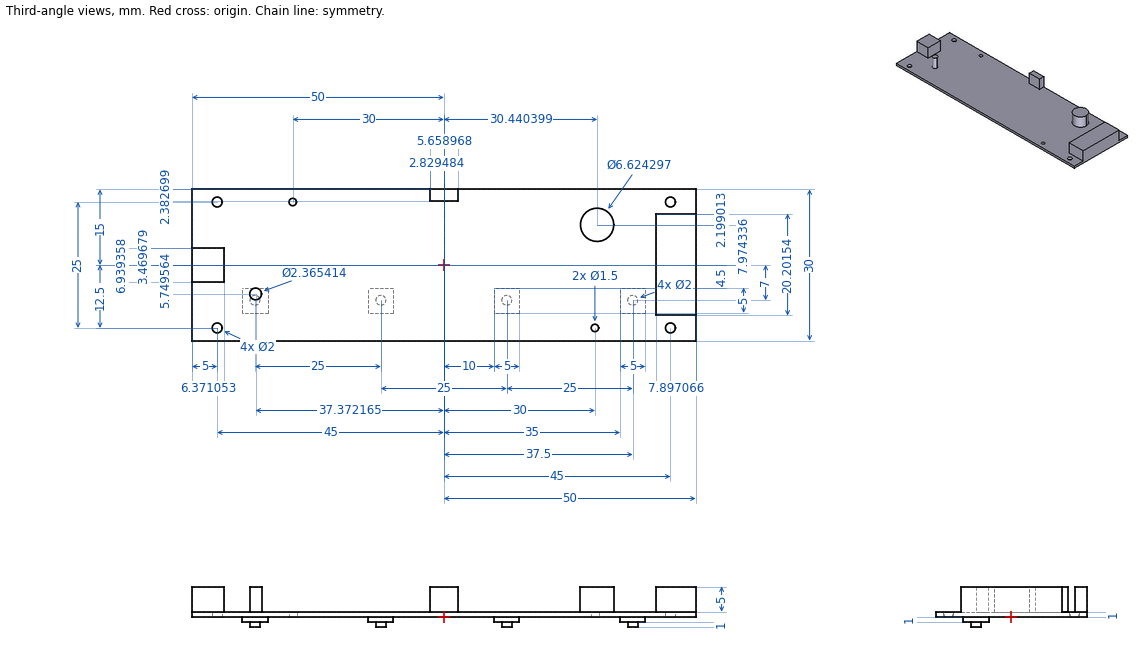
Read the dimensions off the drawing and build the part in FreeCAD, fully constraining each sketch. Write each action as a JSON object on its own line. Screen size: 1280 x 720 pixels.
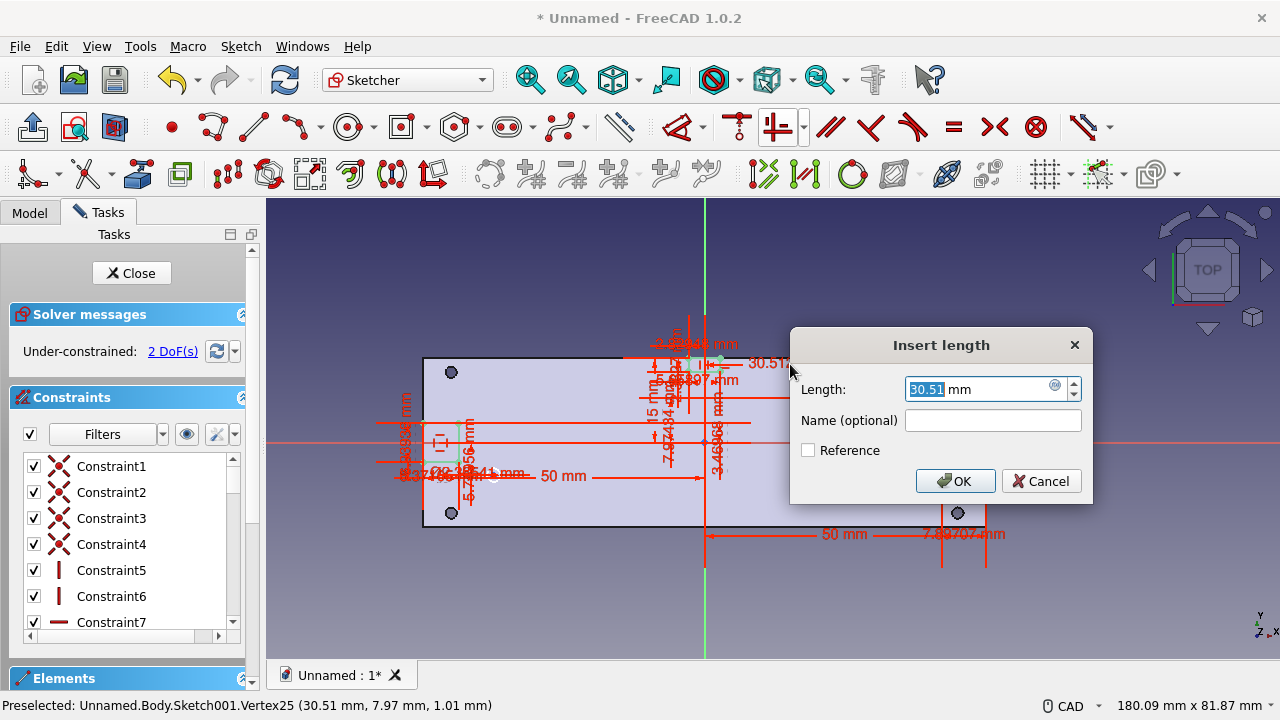
{"action": "type", "text": "30.440399"}
{"action": "key", "text": "Return"}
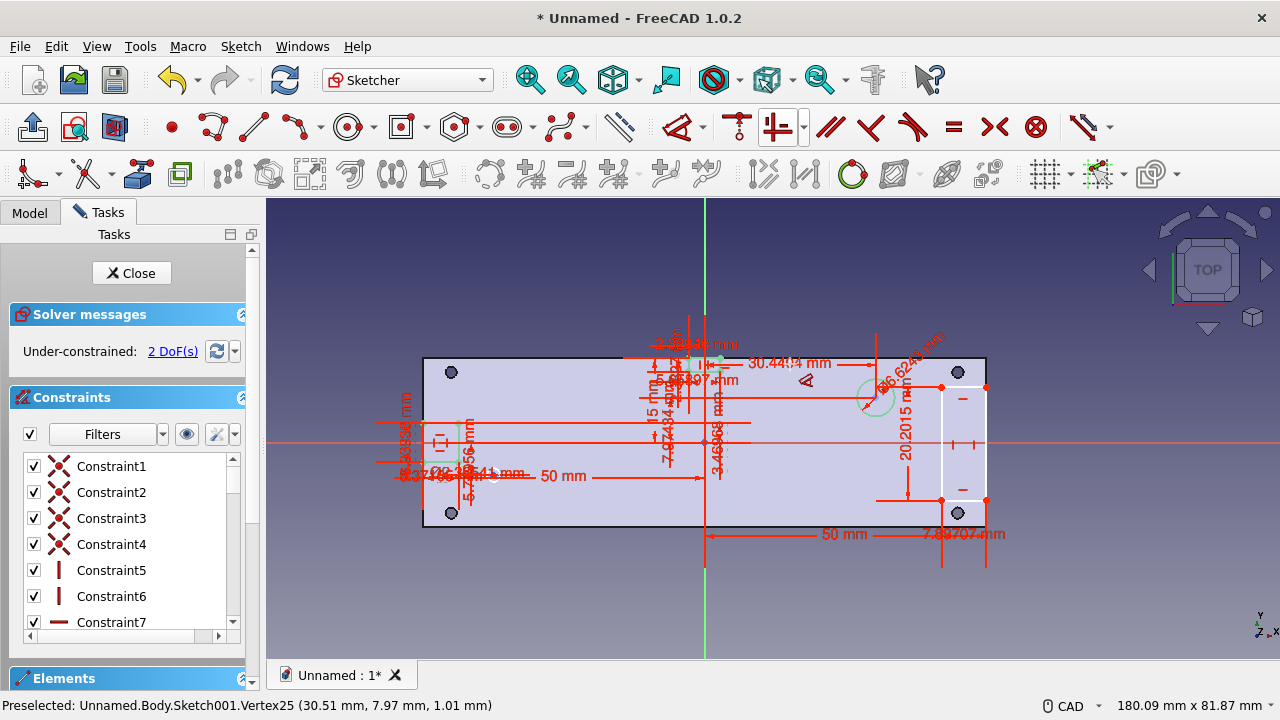
{"action": "left_click", "coordinate": [494, 475]}
{"action": "left_click", "coordinate": [599, 509]}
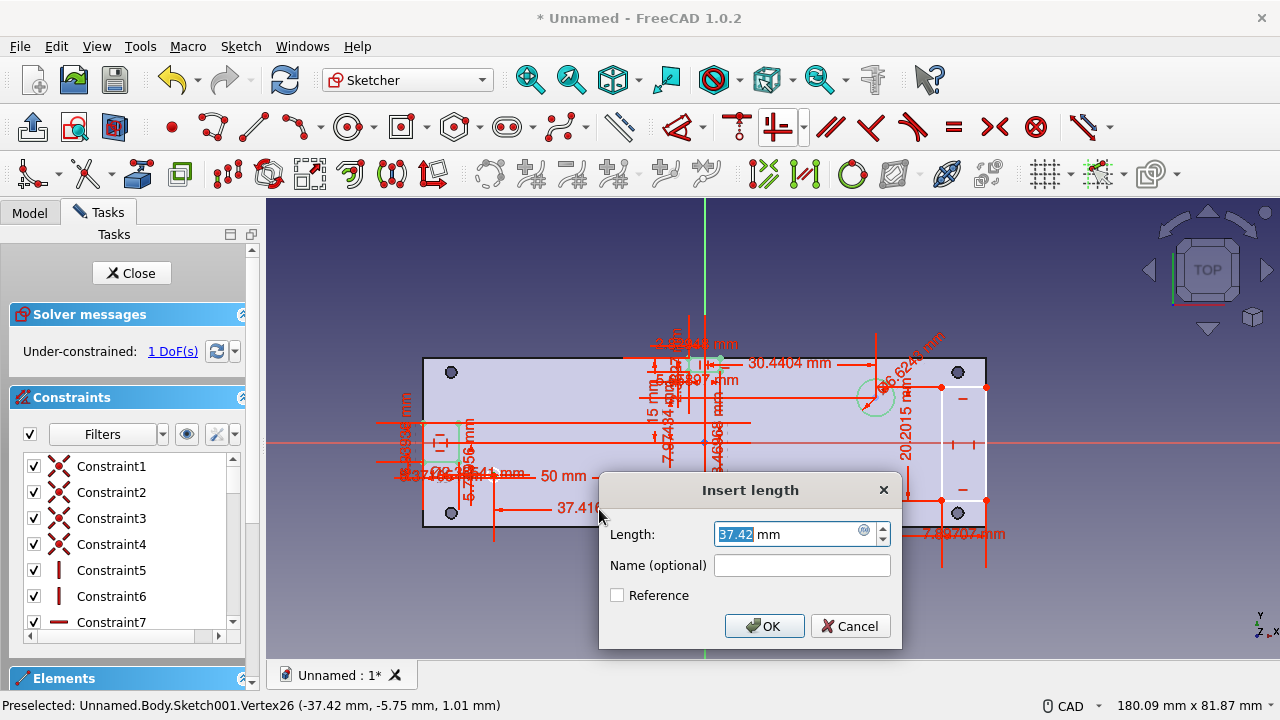
{"action": "type", "text": "37.372165"}
{"action": "key", "text": "Return"}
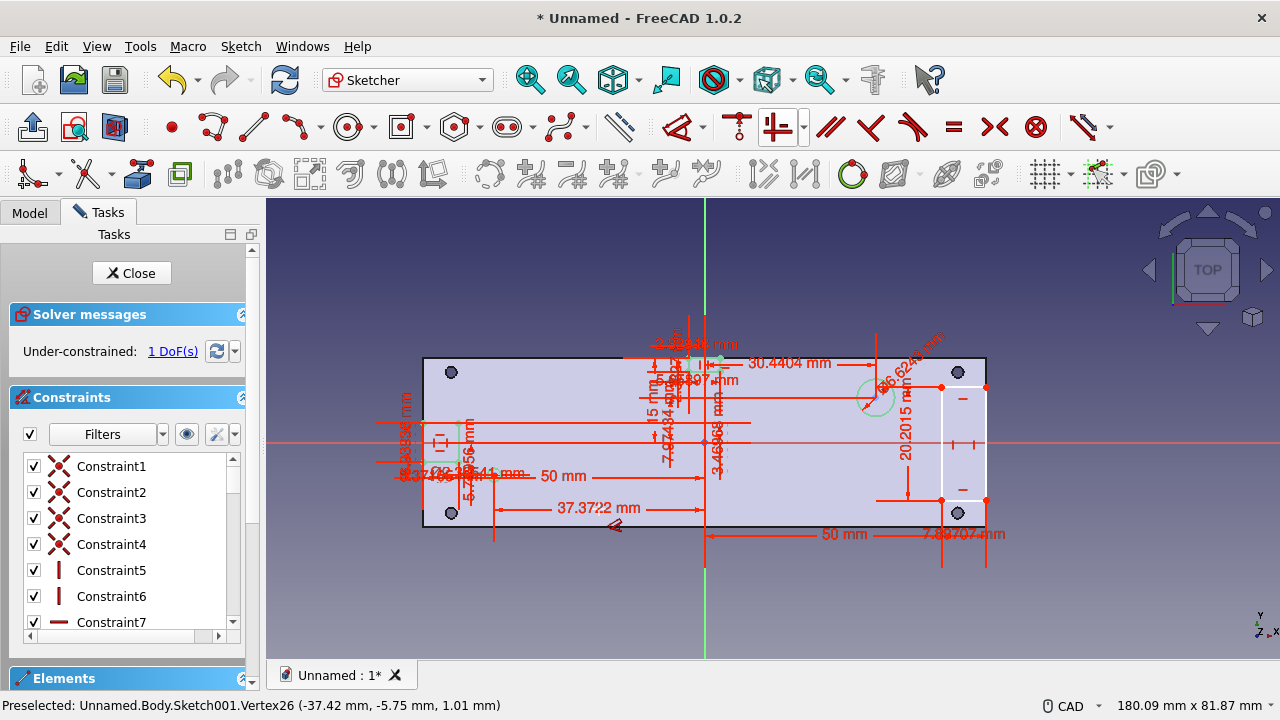
{"action": "scroll", "coordinate": [942, 387], "scroll_direction": "up", "scroll_amount": 6}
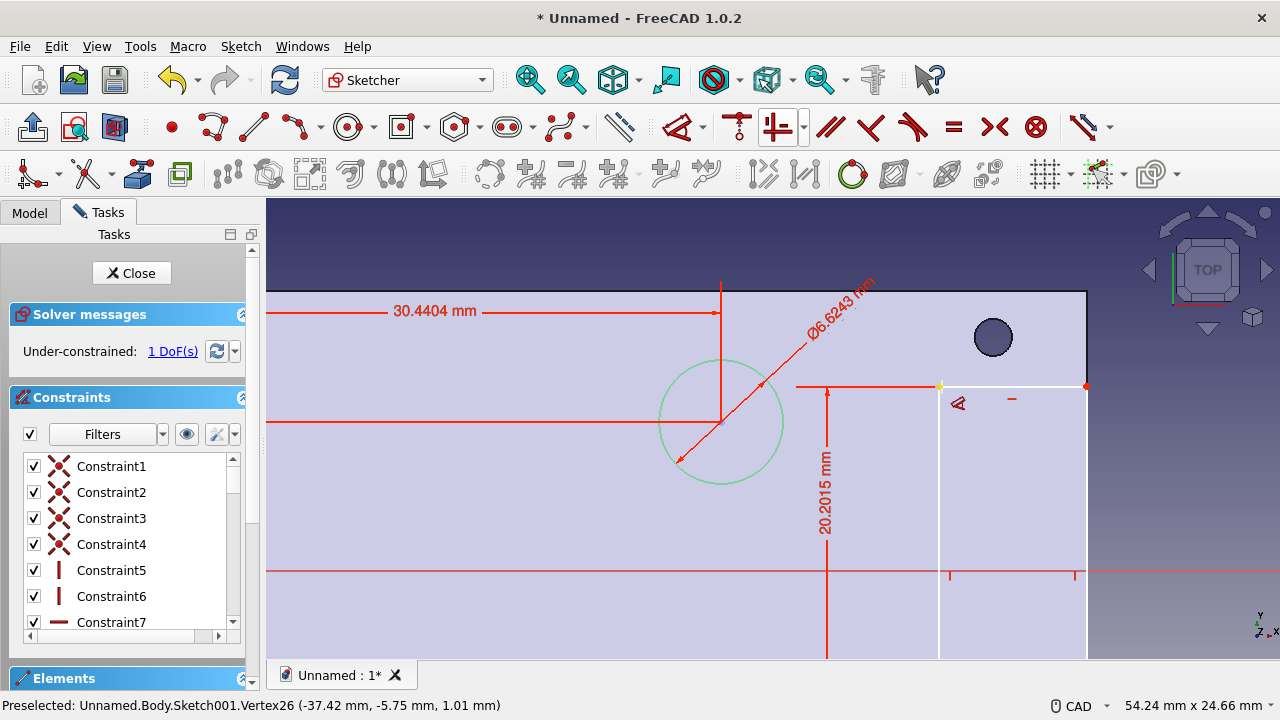
{"action": "left_click", "coordinate": [939, 387]}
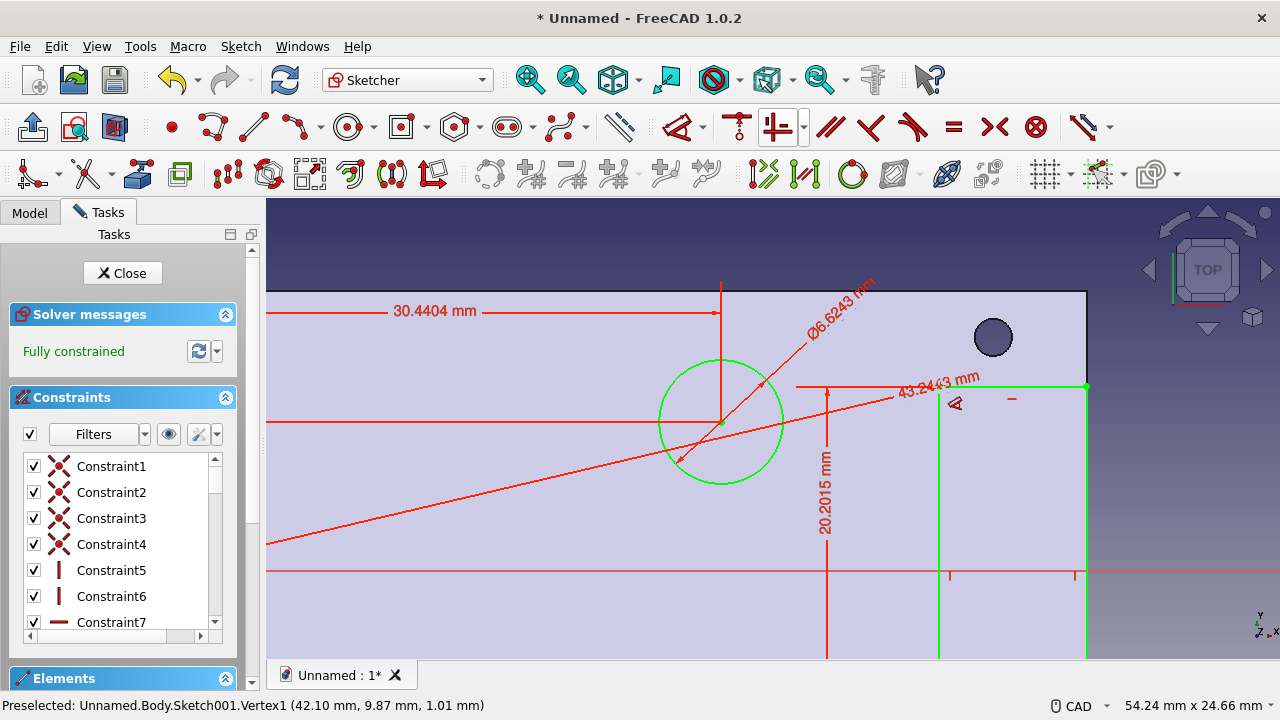
{"action": "left_click", "coordinate": [721, 422]}
{"action": "left_click", "coordinate": [973, 404]}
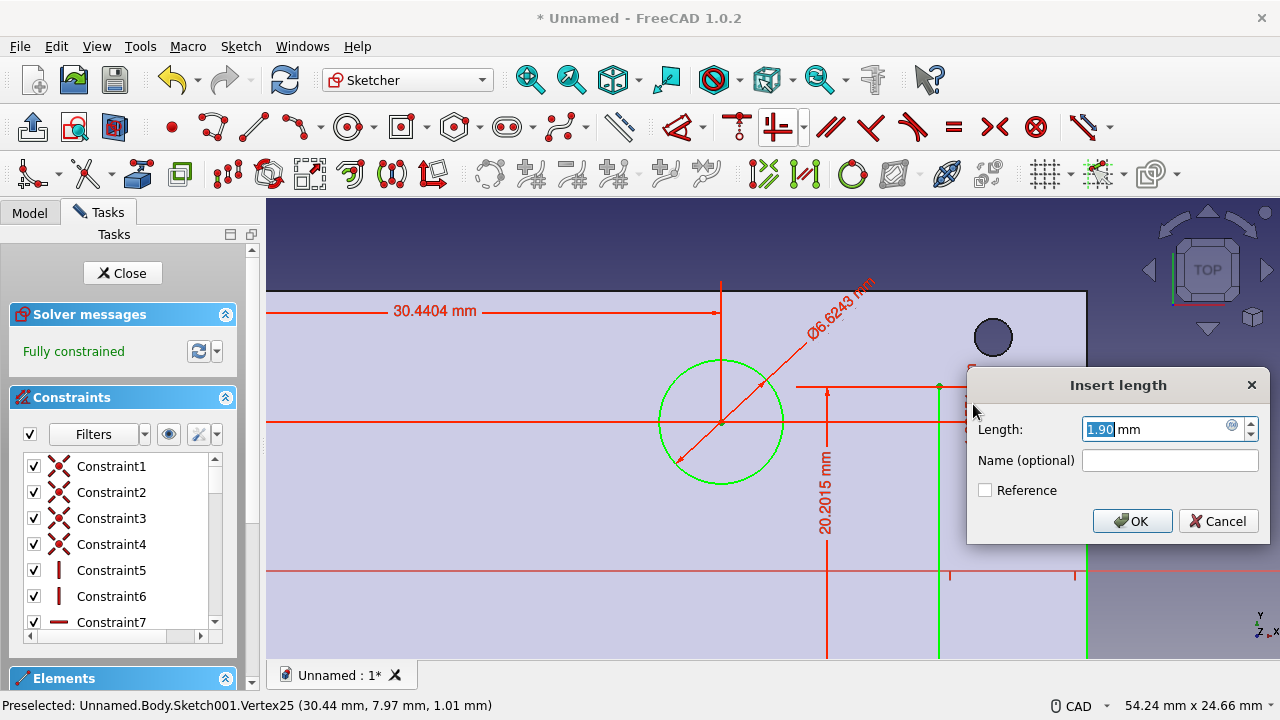
{"action": "type", "text": "2.199013"}
{"action": "key", "text": "Return"}
{"action": "key", "text": "Escape"}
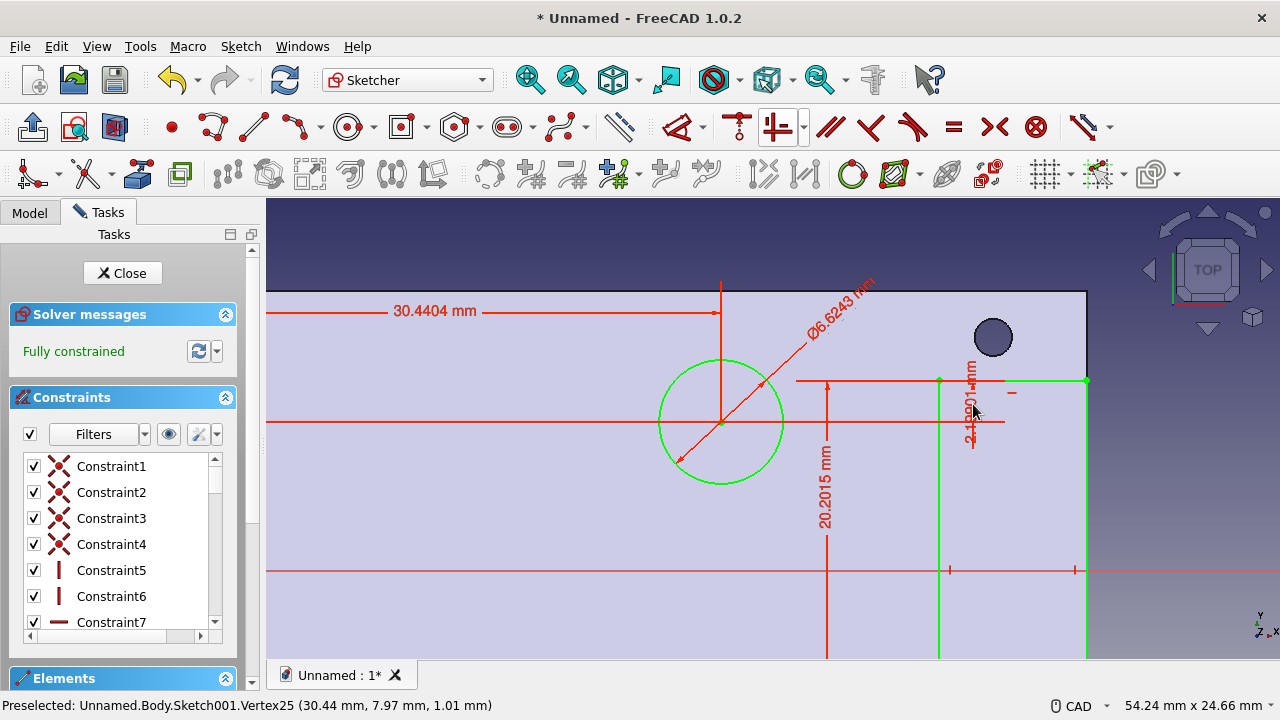
{"action": "left_click", "coordinate": [123, 273]}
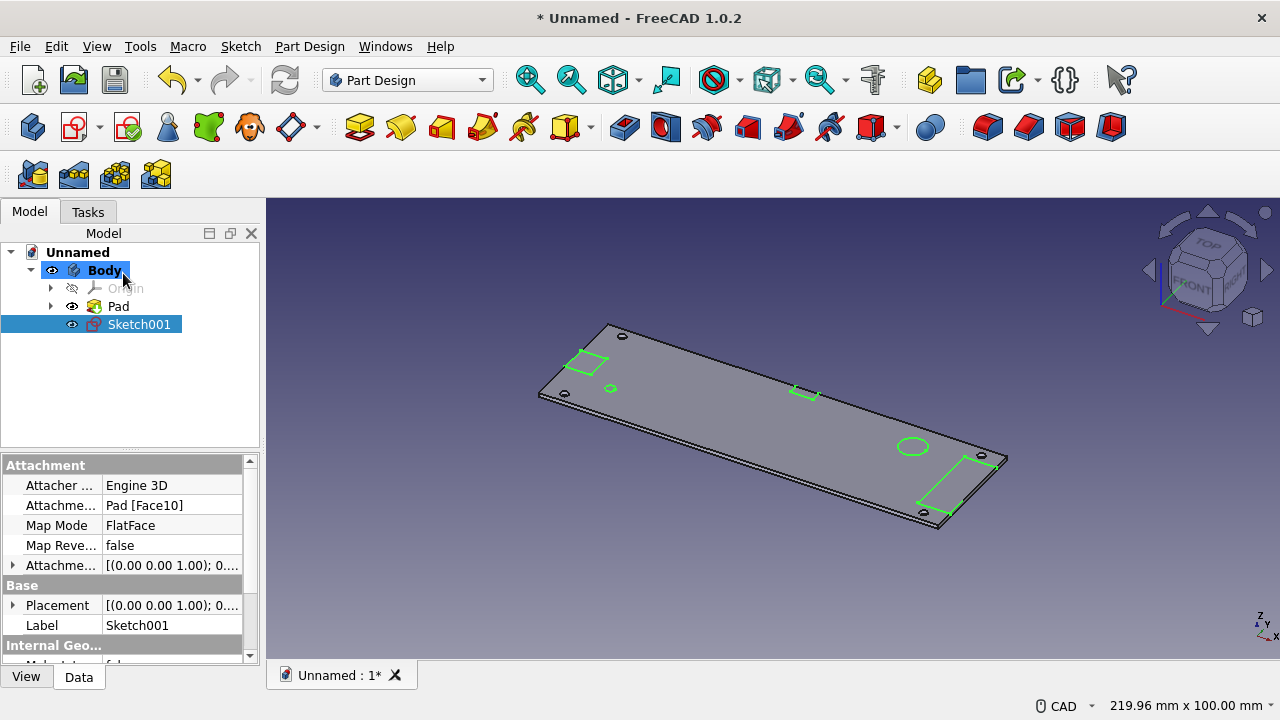
{"action": "left_click", "coordinate": [360, 128]}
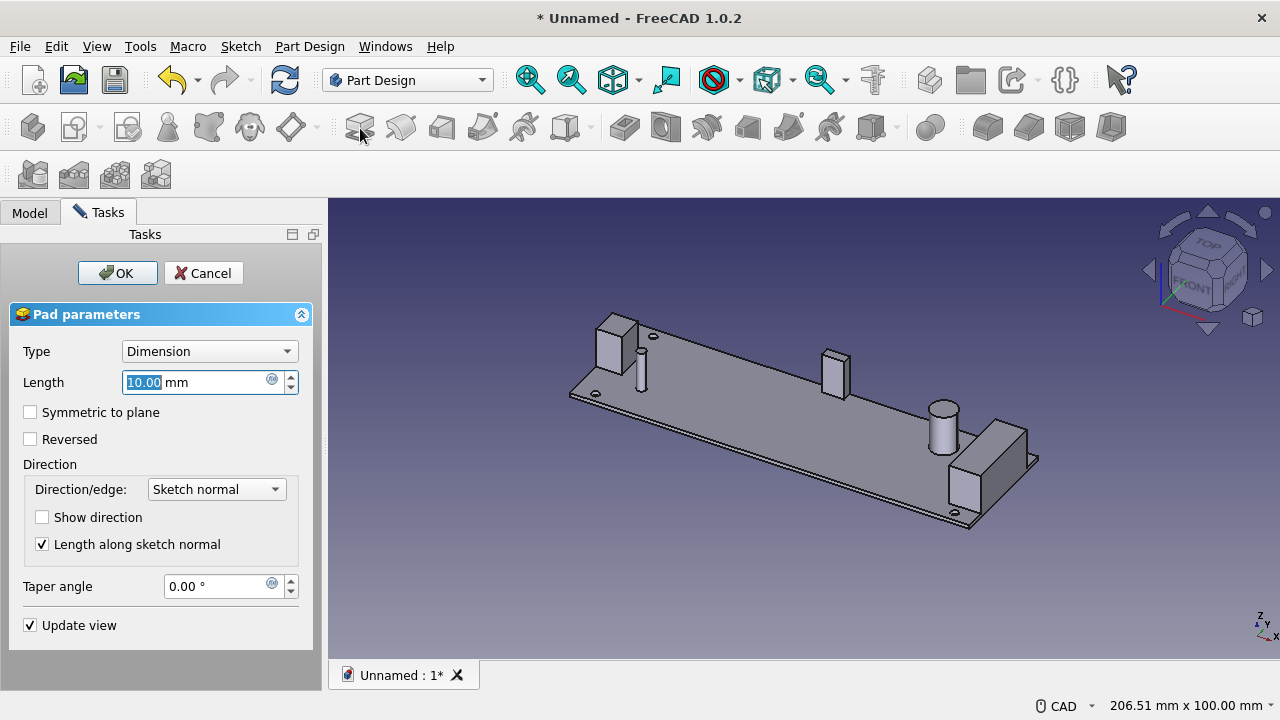
{"action": "type", "text": "5"}
{"action": "key", "text": "Tab"}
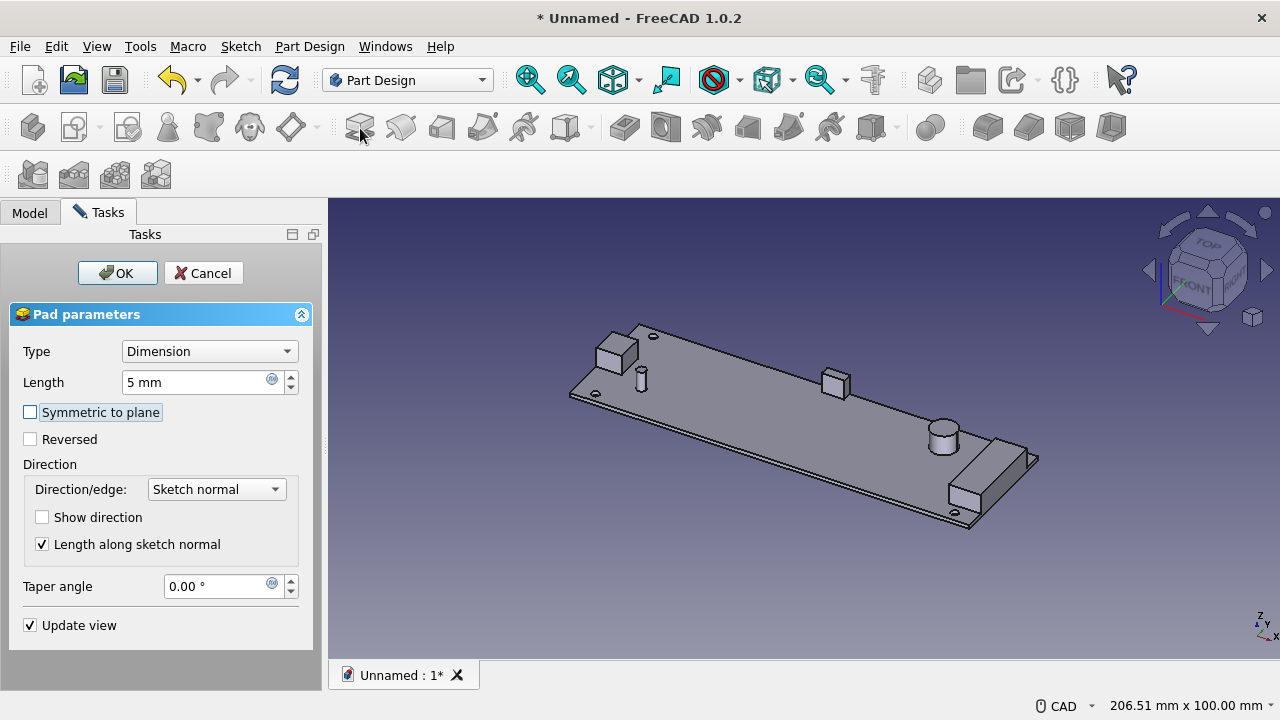
{"action": "left_click", "coordinate": [118, 273]}